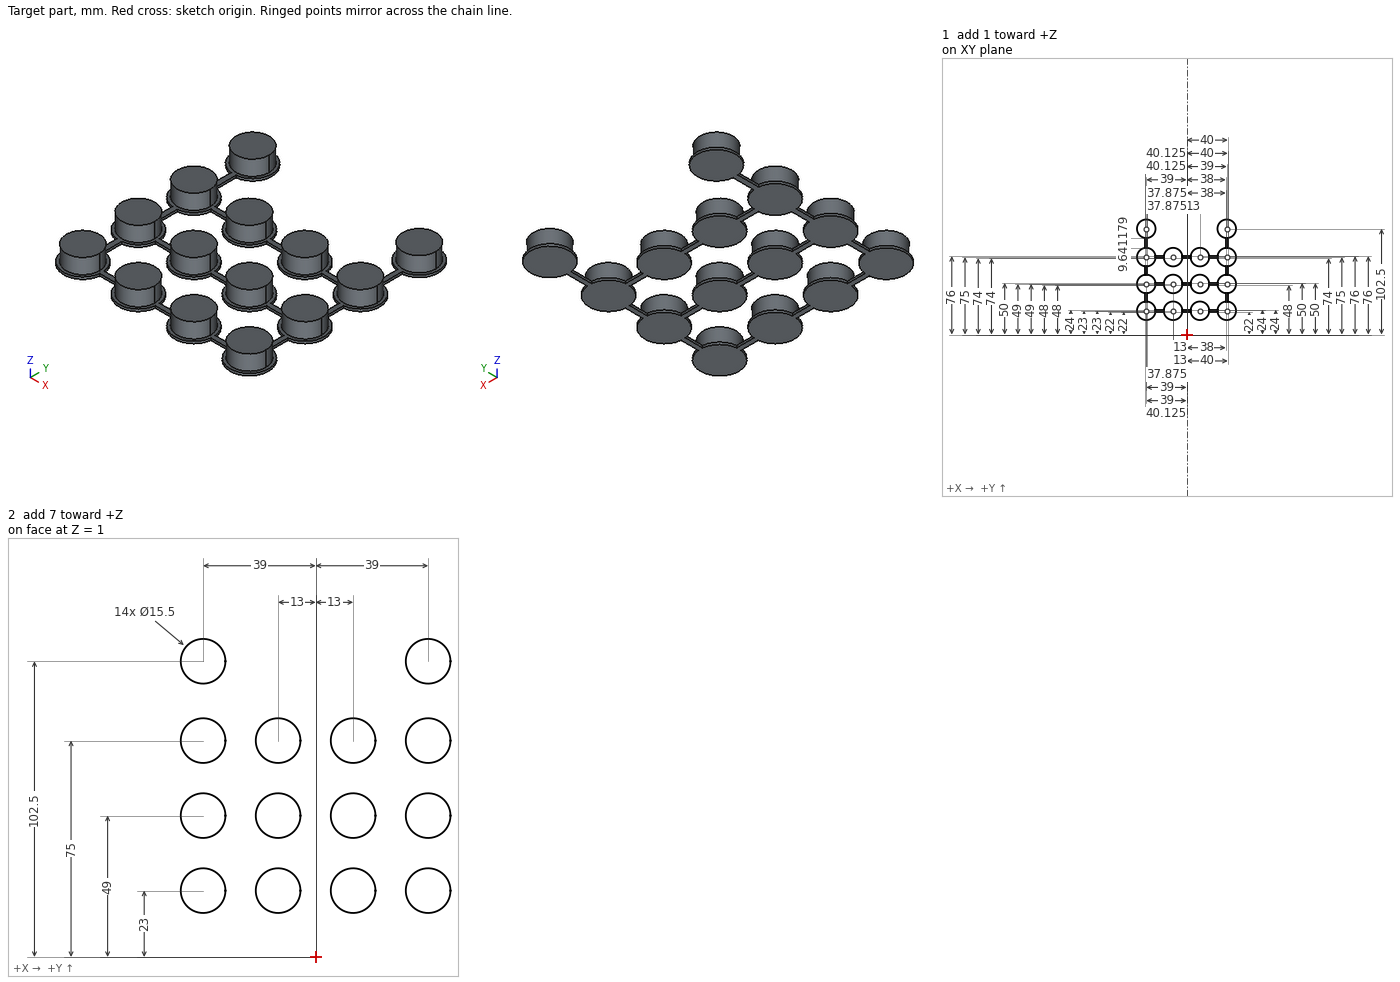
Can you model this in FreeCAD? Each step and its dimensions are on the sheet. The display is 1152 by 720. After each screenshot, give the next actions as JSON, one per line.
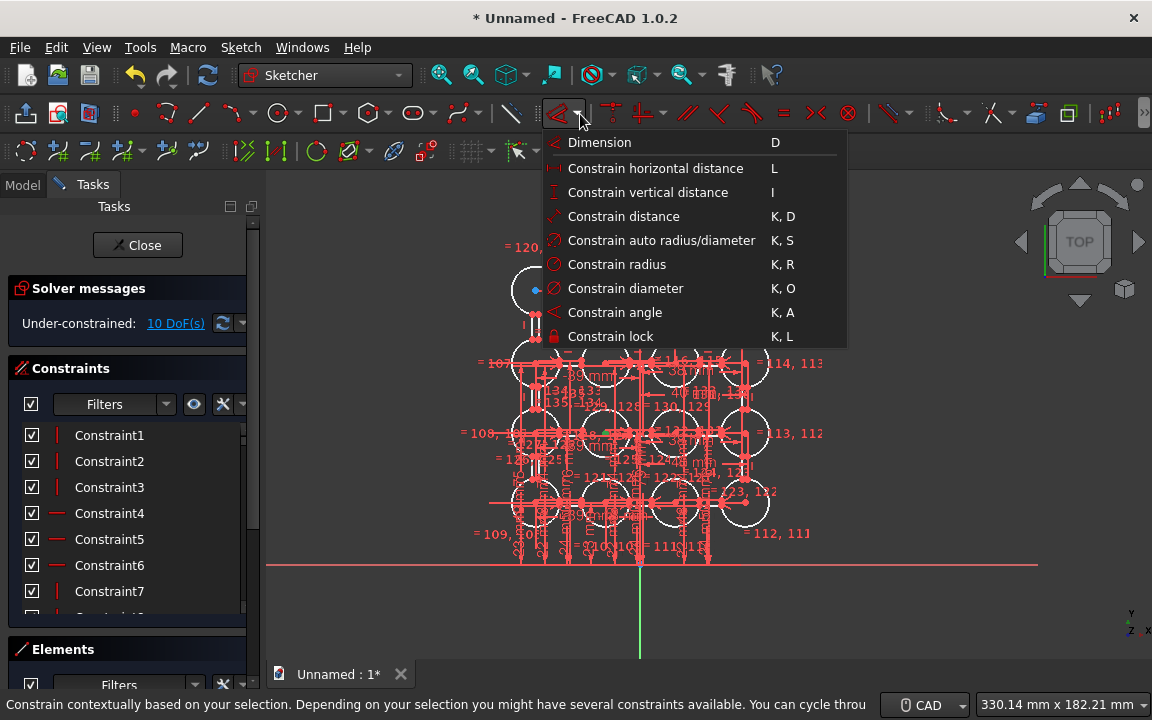
{"action": "left_click", "coordinate": [695, 168]}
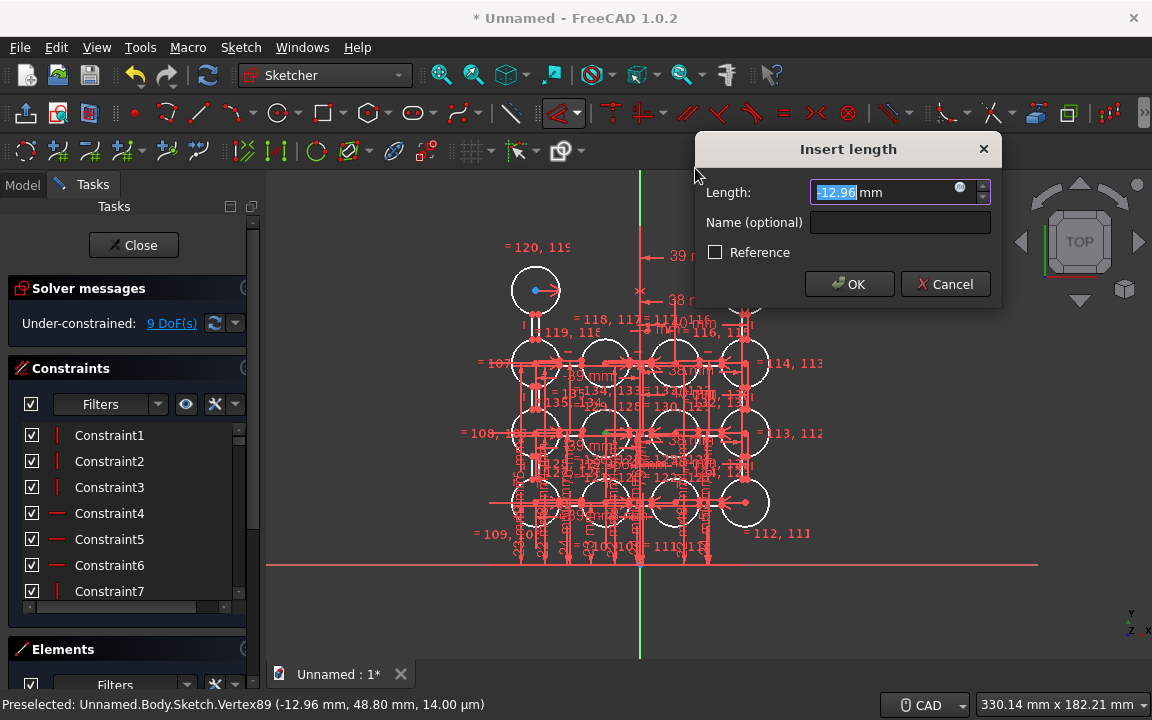
{"action": "type", "text": "-13"}
{"action": "key", "text": "Return"}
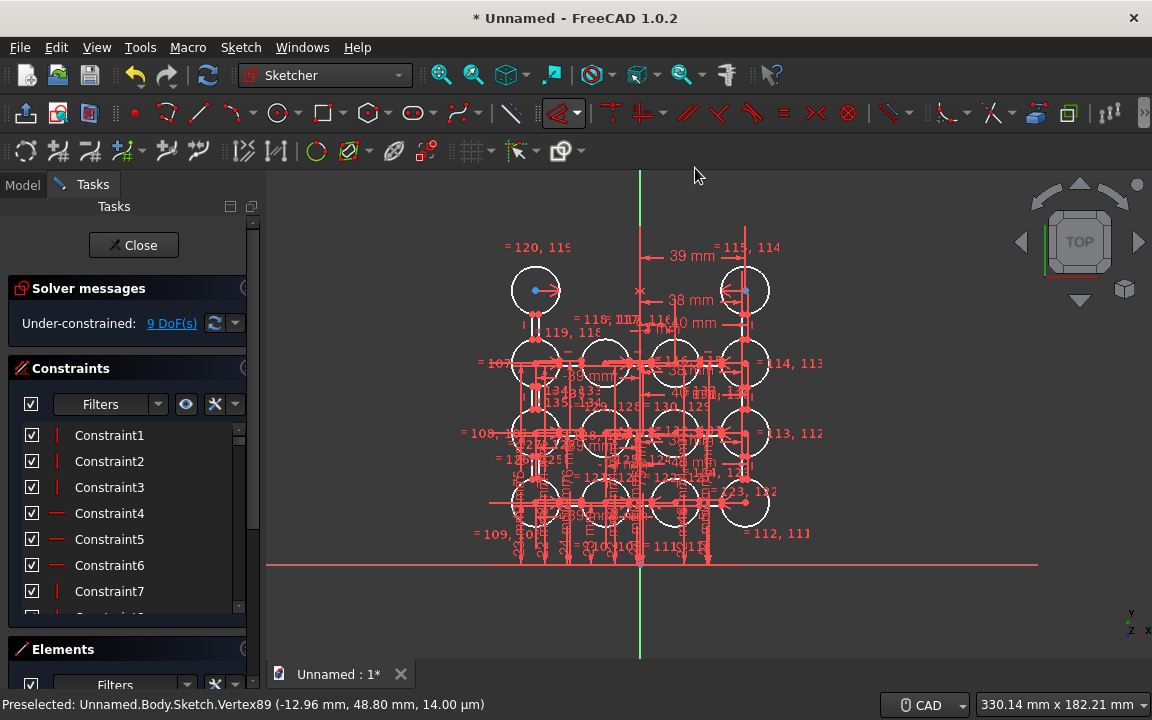
{"action": "left_click", "coordinate": [606, 434]}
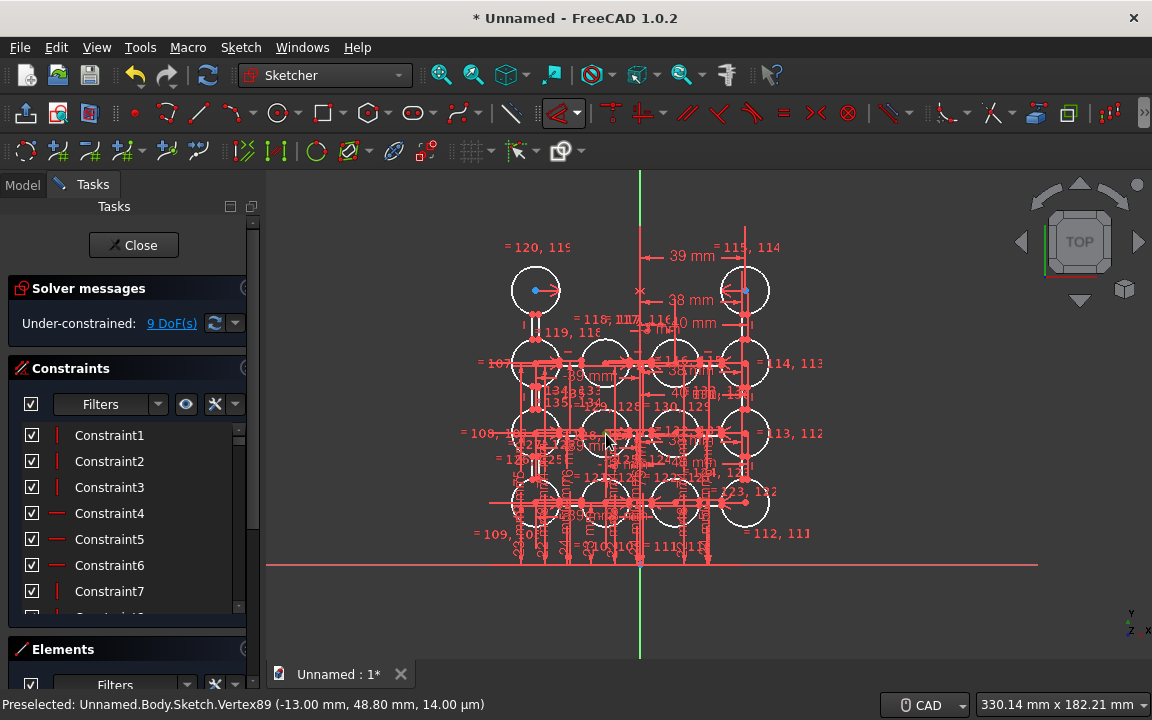
{"action": "left_click", "coordinate": [580, 114]}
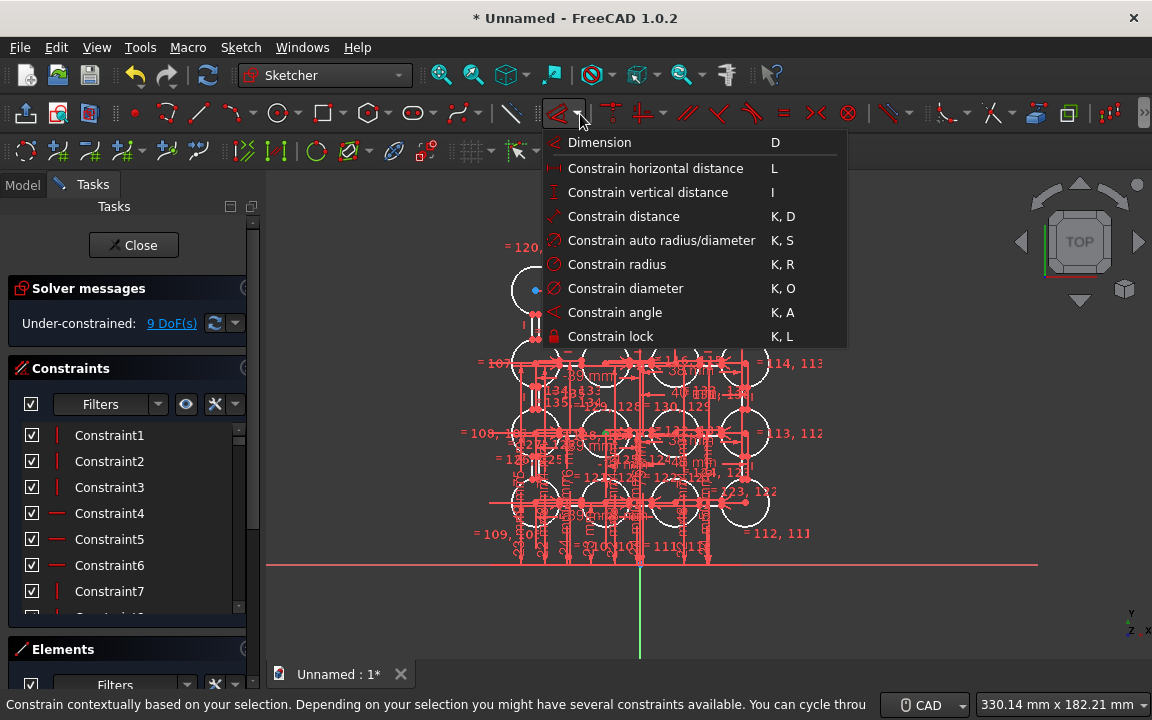
{"action": "left_click", "coordinate": [695, 192]}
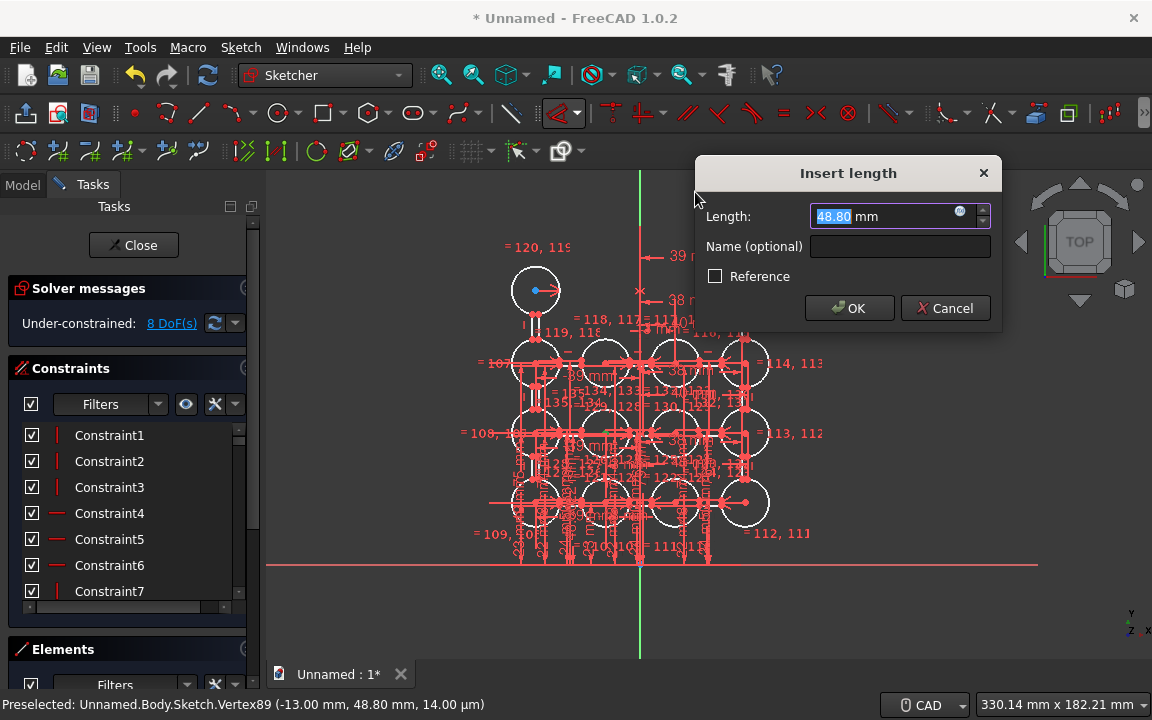
{"action": "type", "text": "49"}
{"action": "key", "text": "Return"}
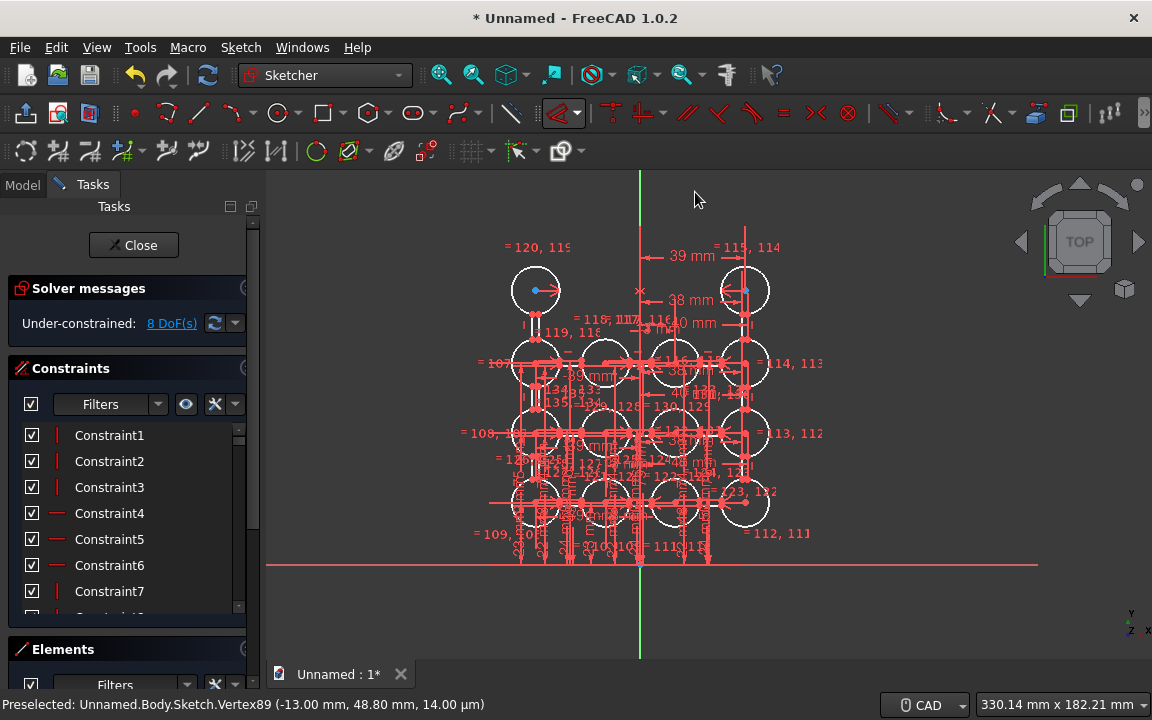
{"action": "left_click", "coordinate": [745, 291]}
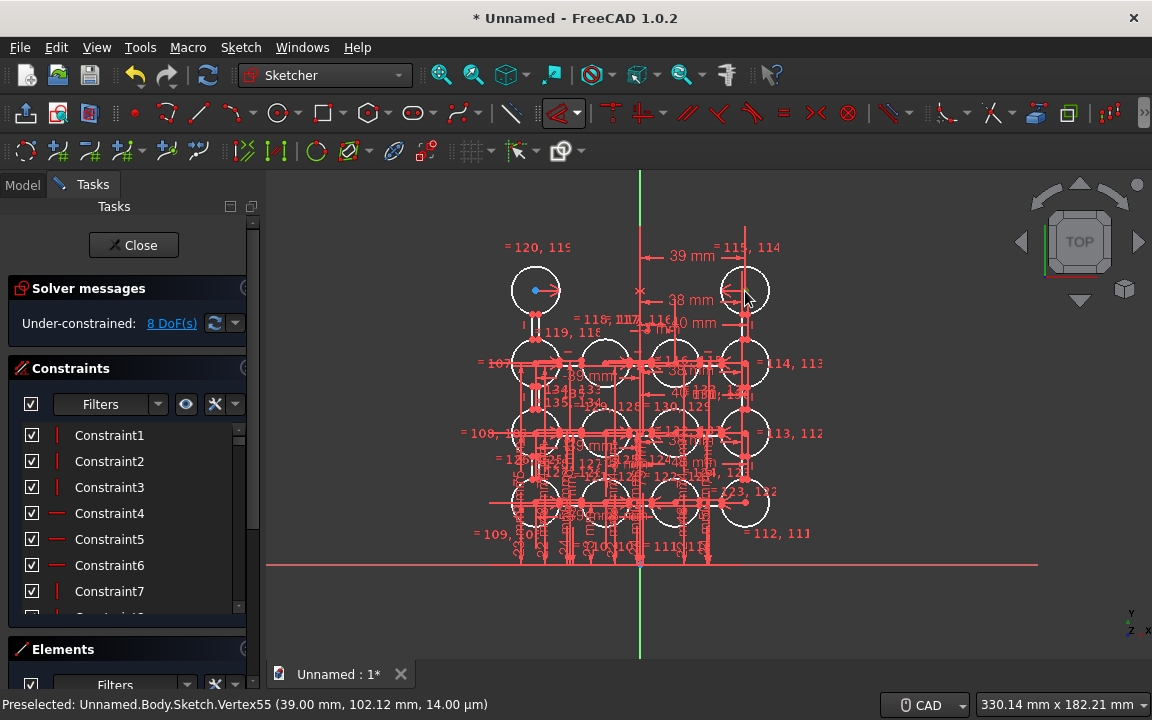
{"action": "left_click", "coordinate": [580, 114]}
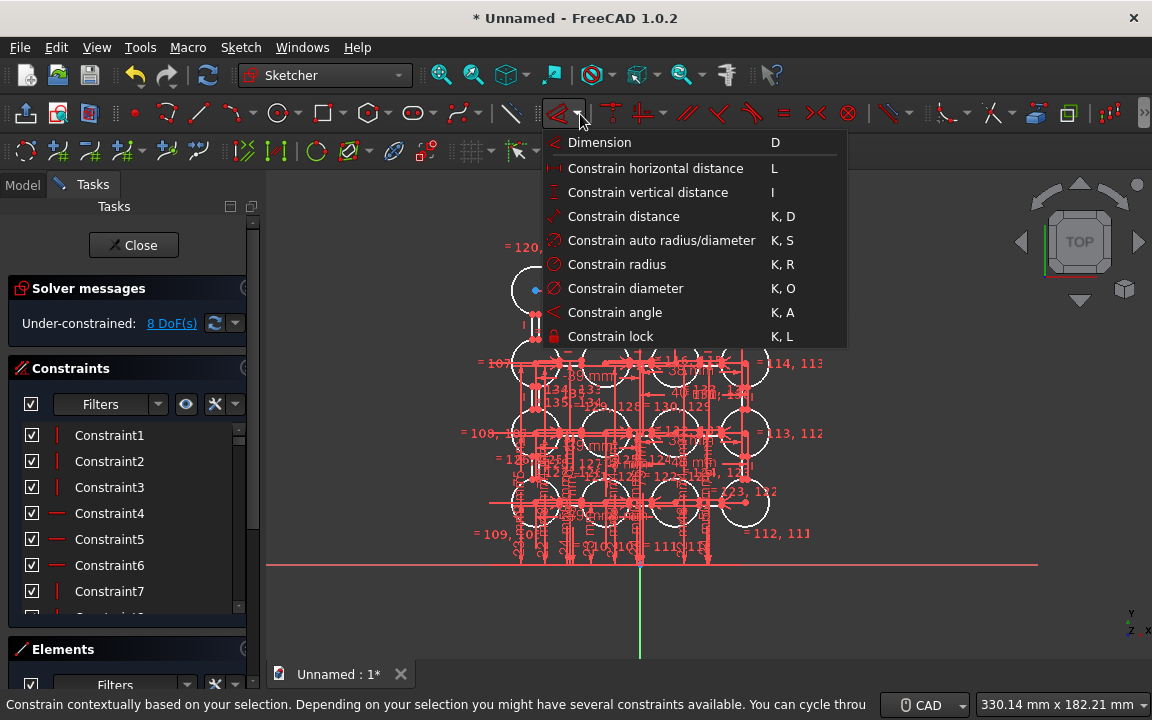
{"action": "left_click", "coordinate": [695, 192]}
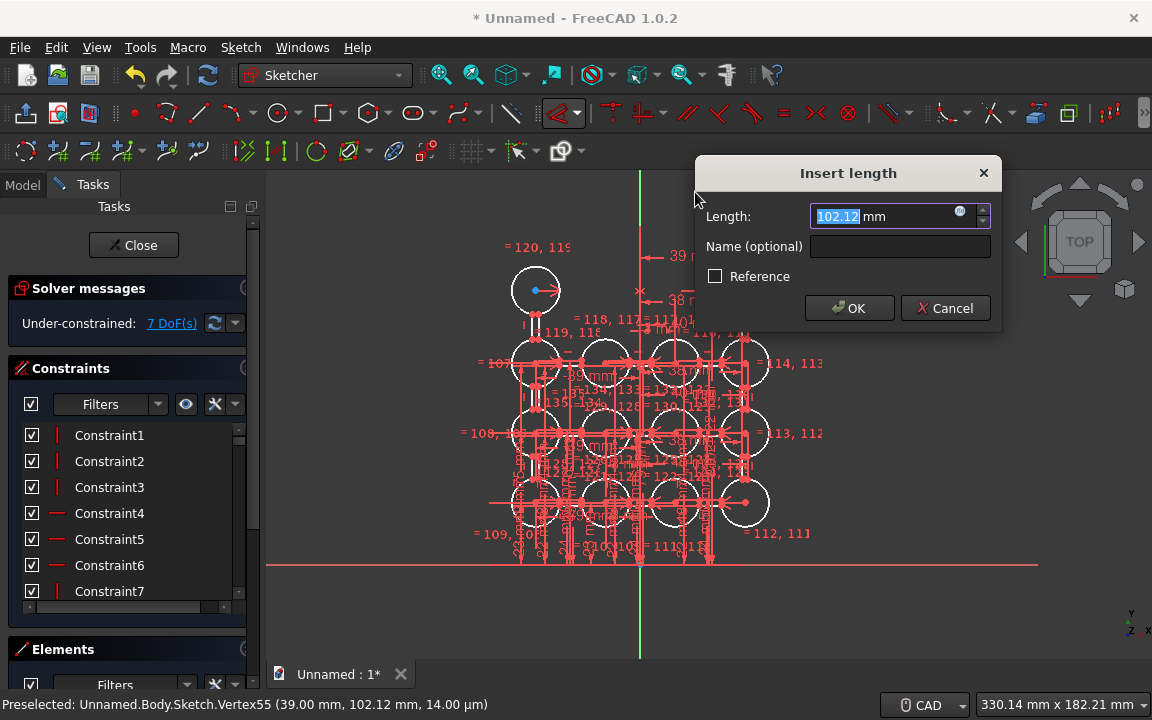
{"action": "type", "text": "102.5"}
{"action": "key", "text": "Return"}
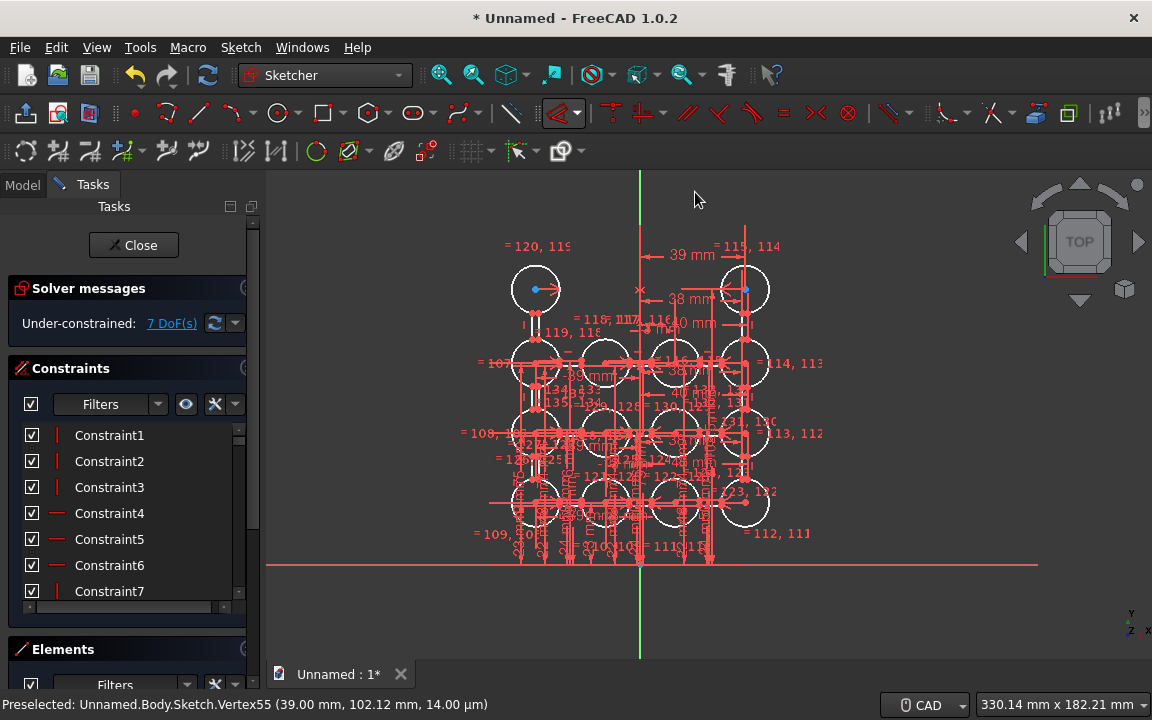
{"action": "scroll", "coordinate": [532, 313], "scroll_direction": "up", "scroll_amount": 4}